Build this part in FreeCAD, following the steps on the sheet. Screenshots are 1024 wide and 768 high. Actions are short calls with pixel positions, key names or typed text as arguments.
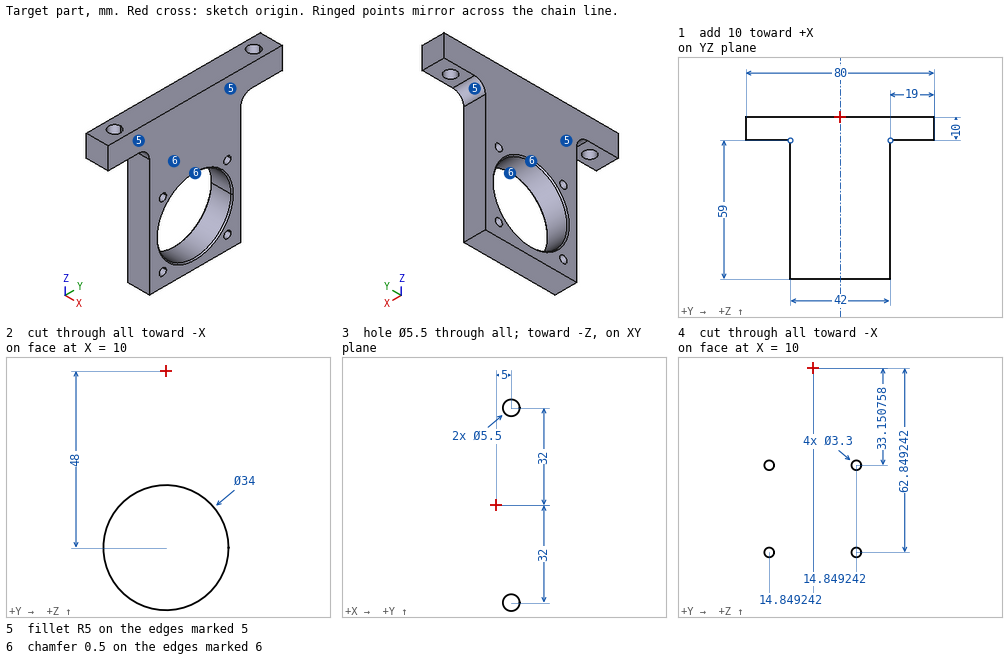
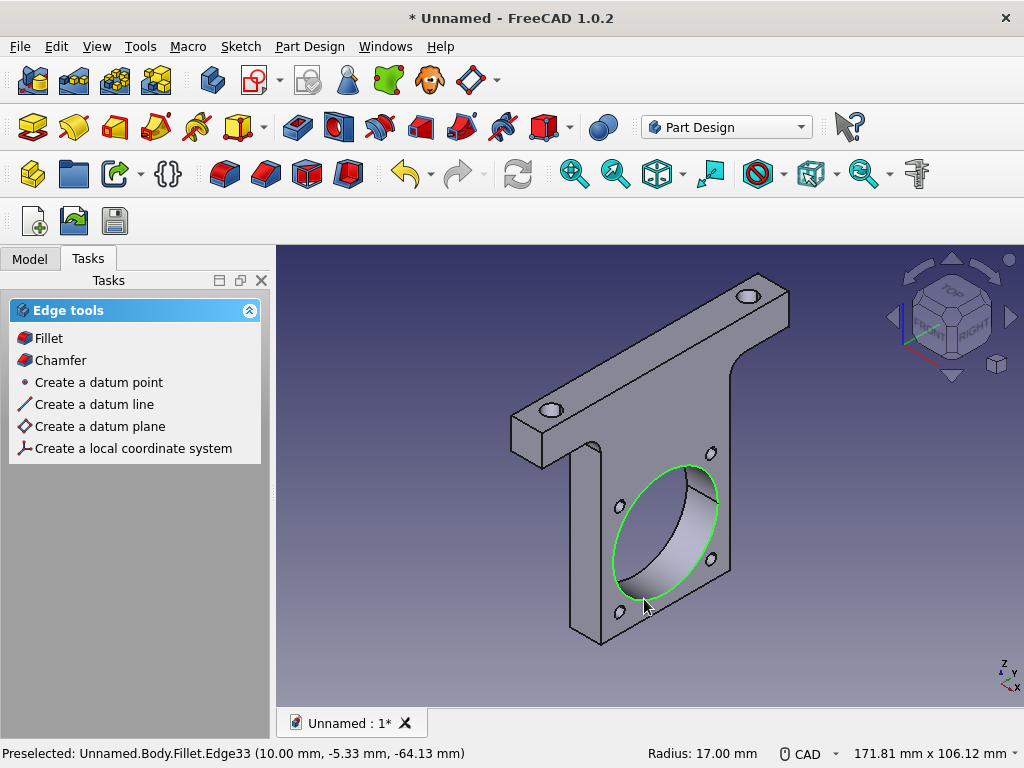
key(2)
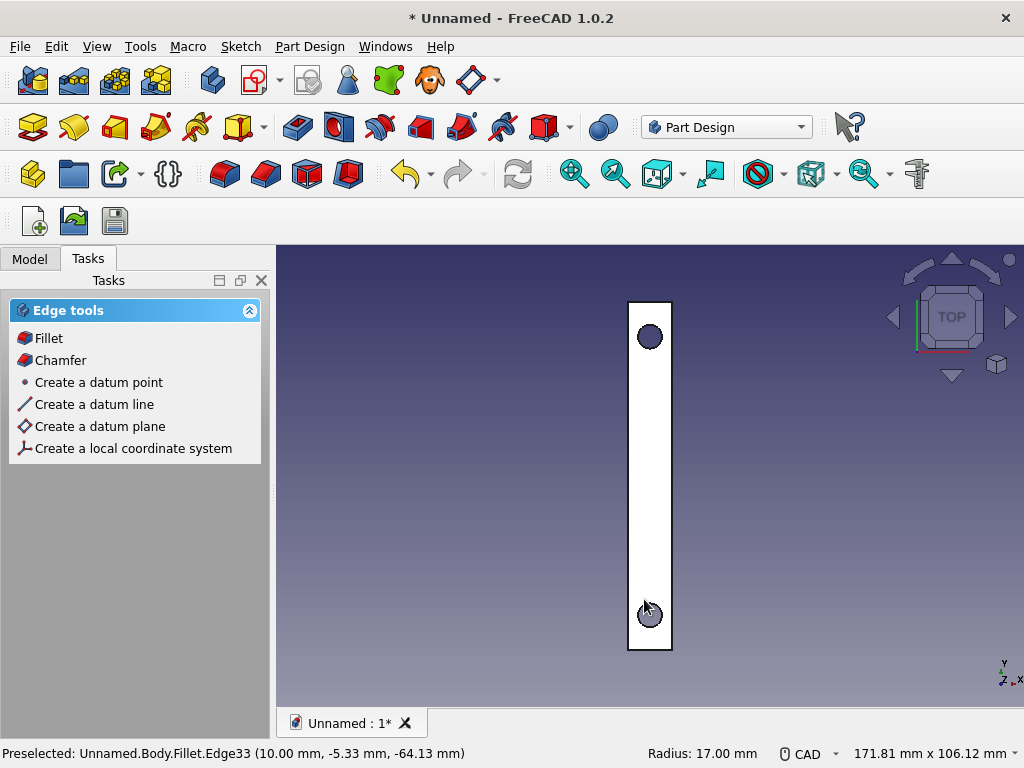
key(0)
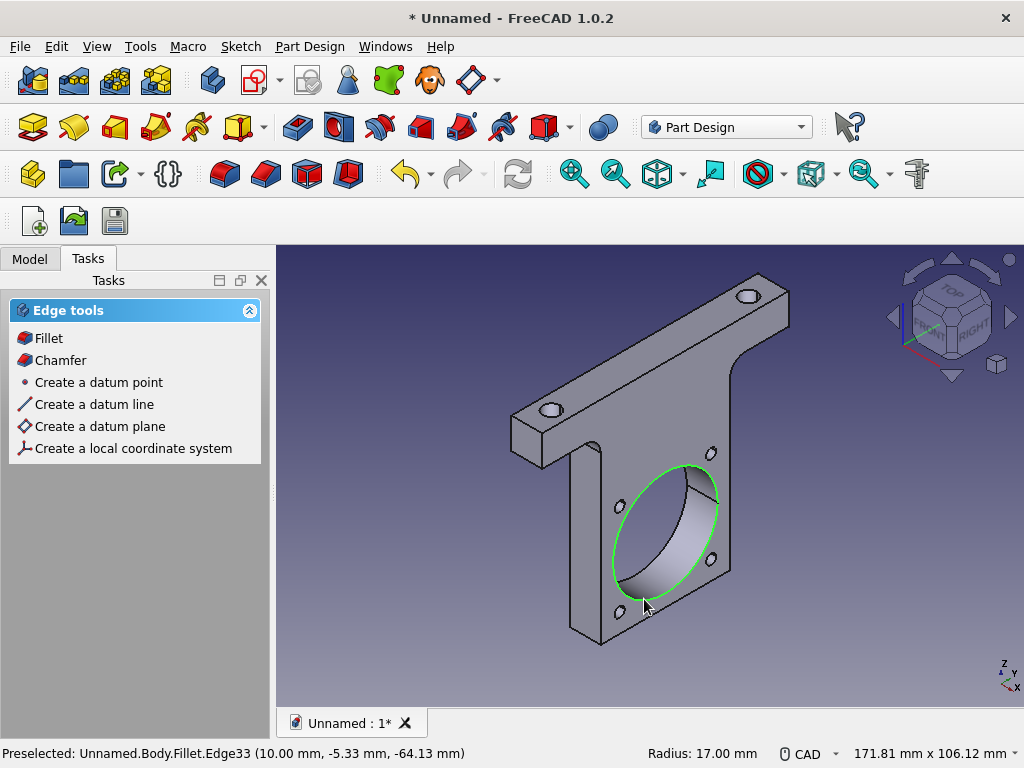
key(1)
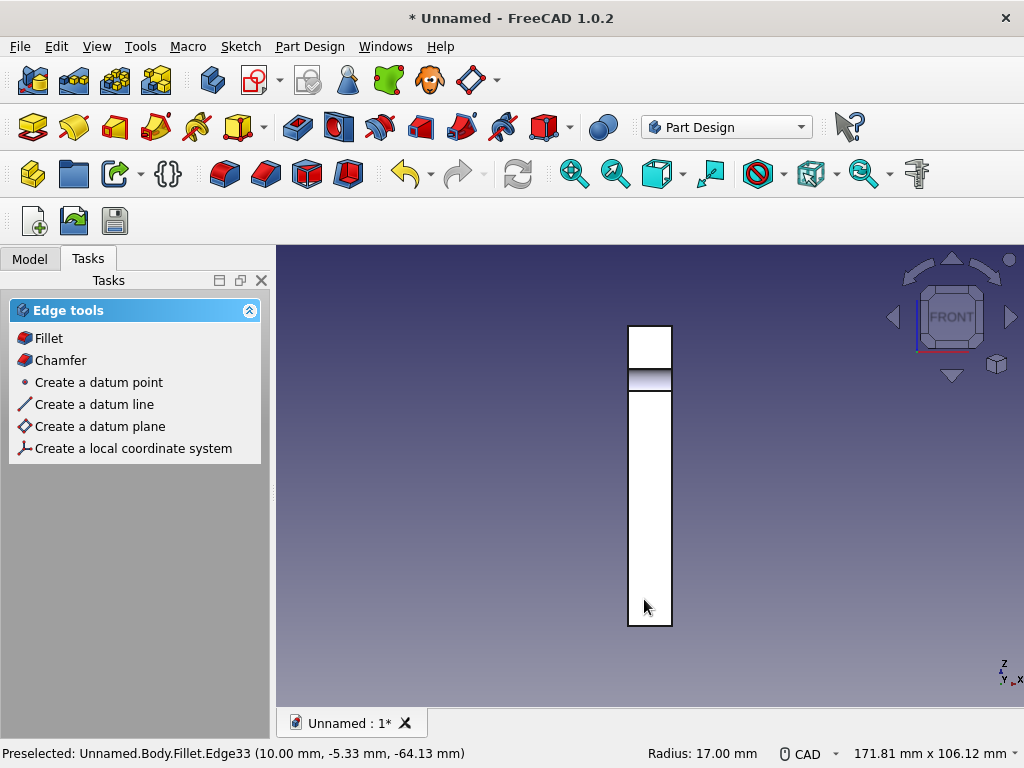
key(3)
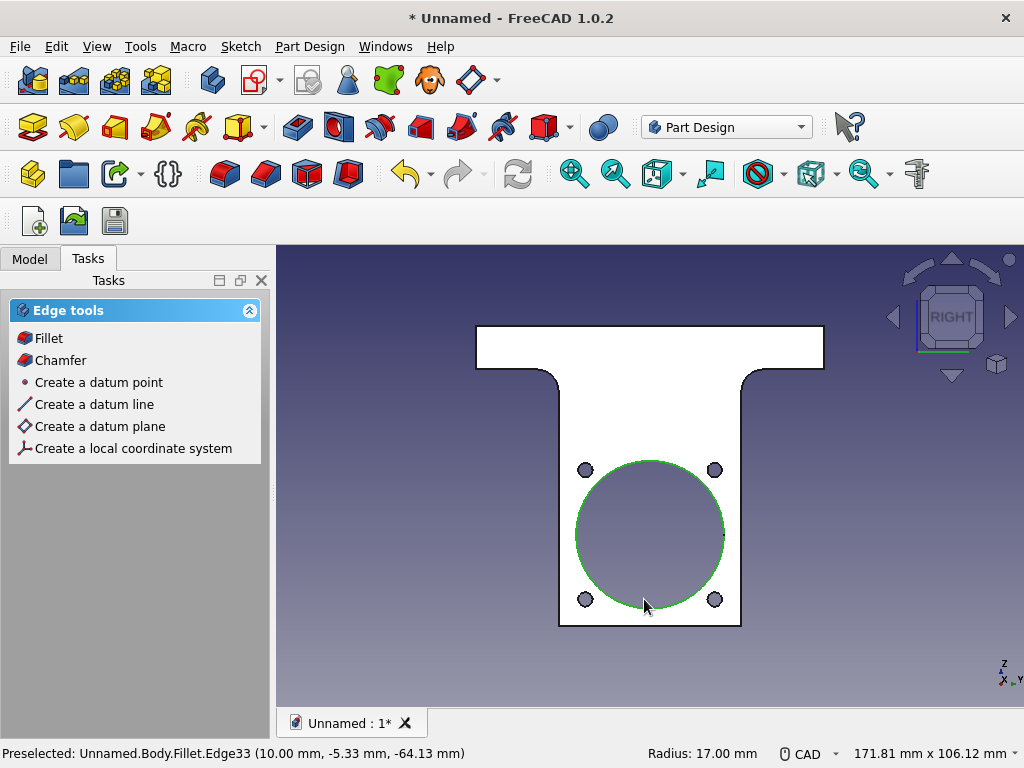
key(5)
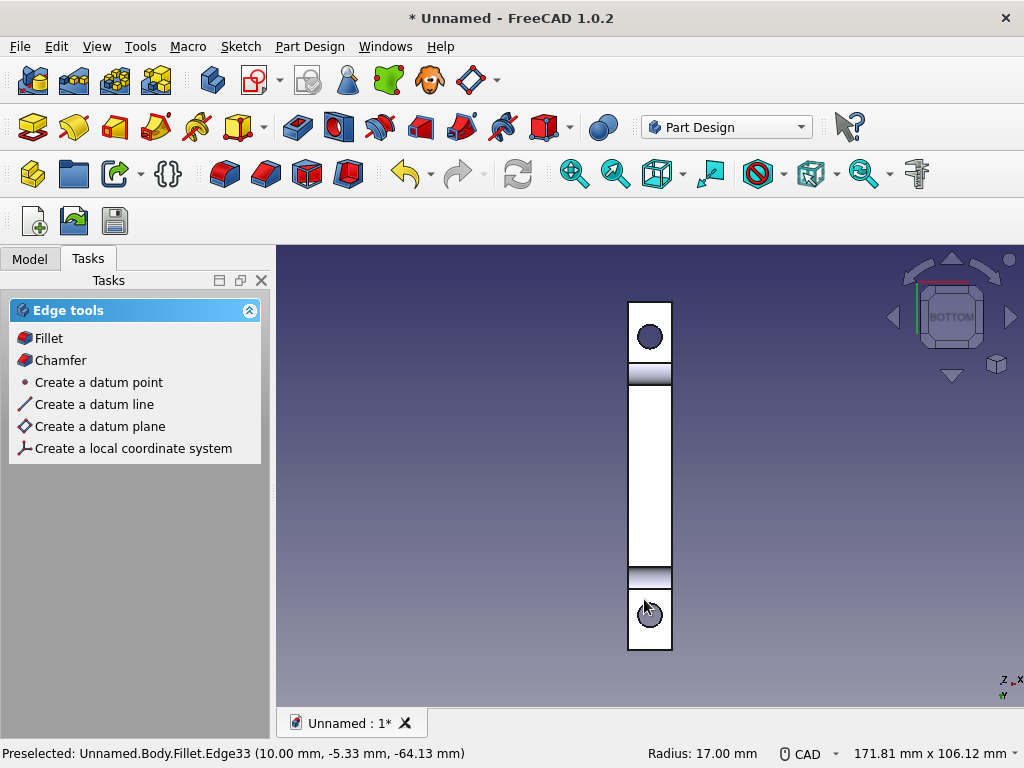
key(4)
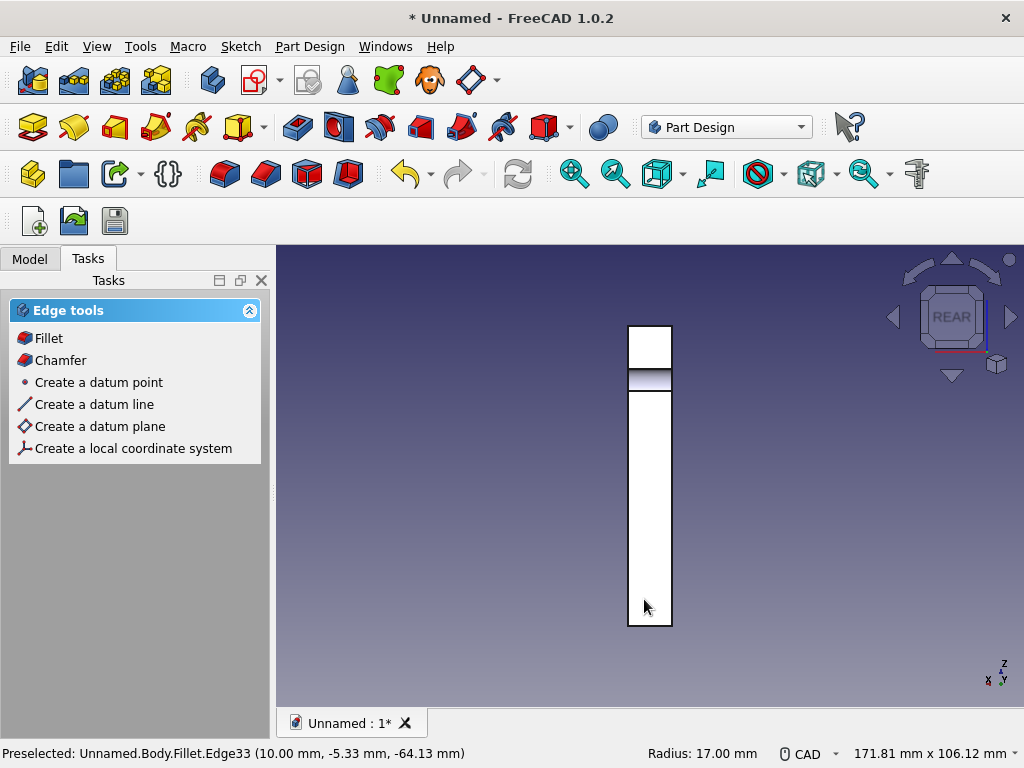
key(6)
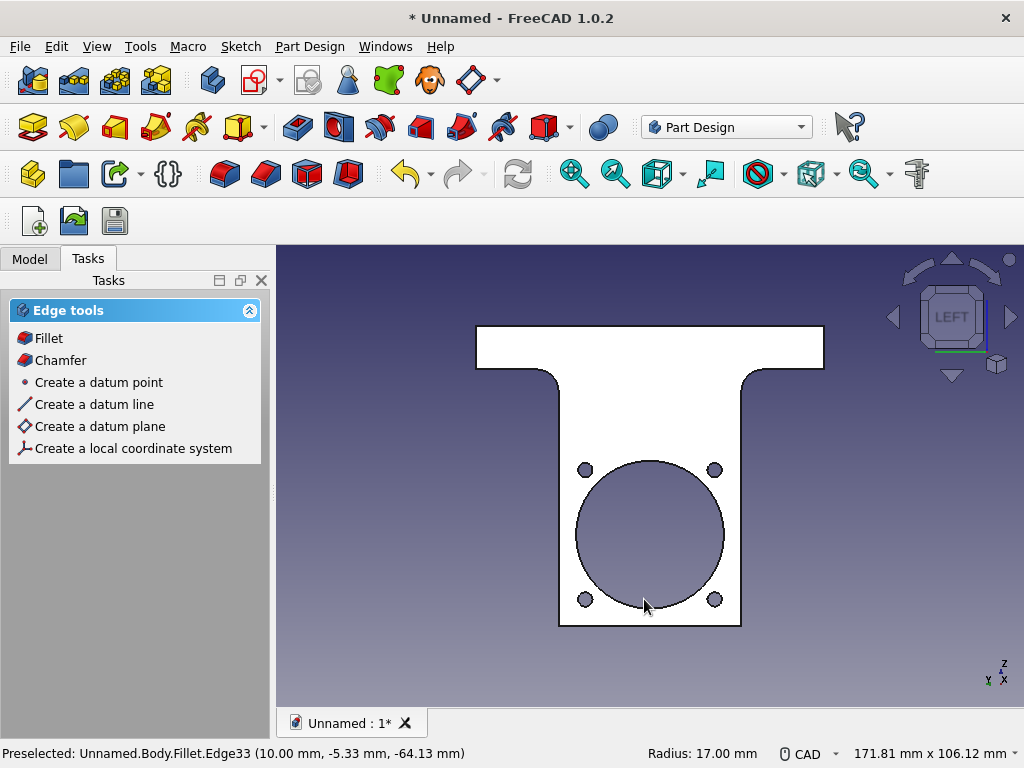
click(724, 534, ctrl)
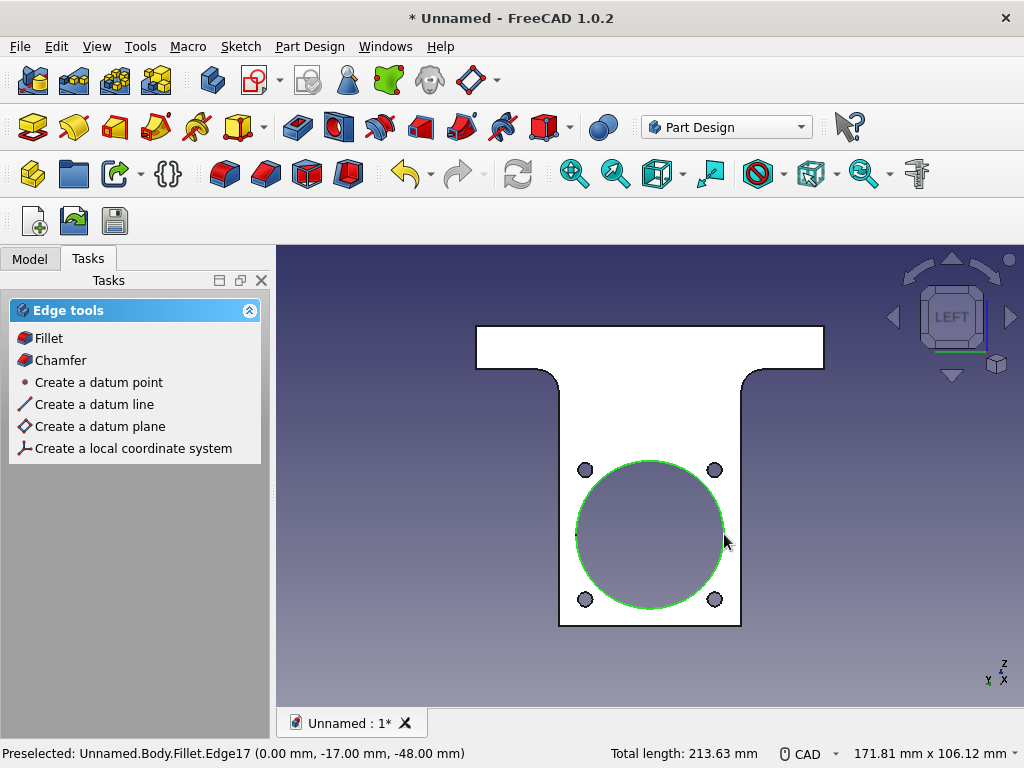
click(266, 174)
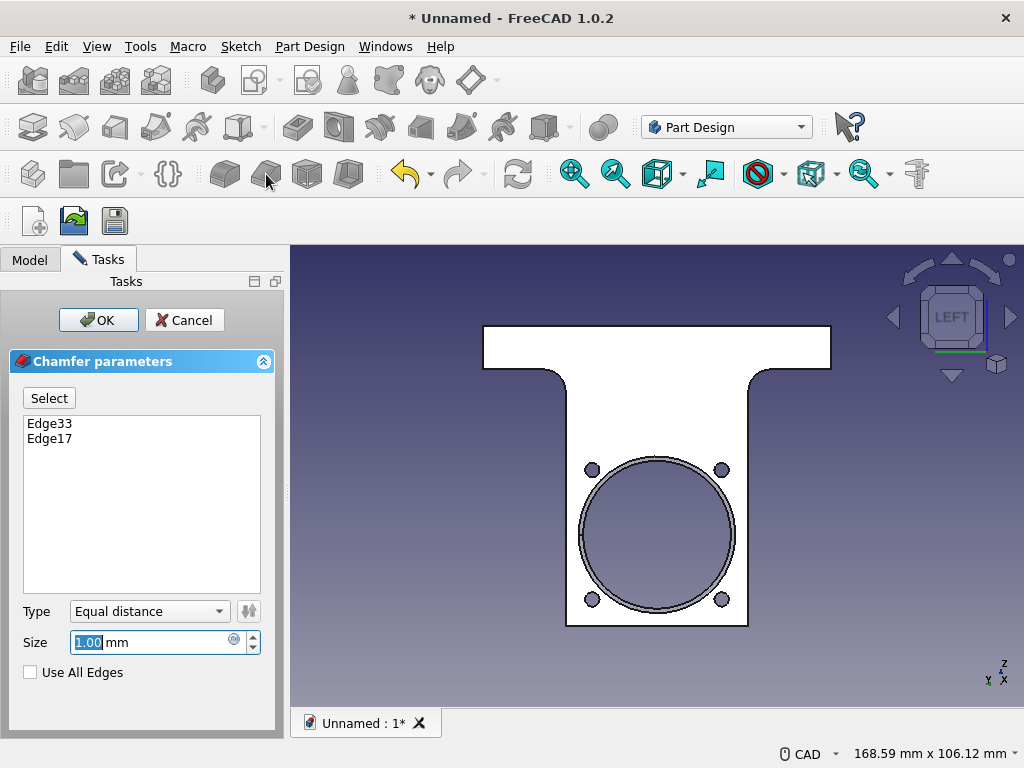
text(0.5)
key(Tab)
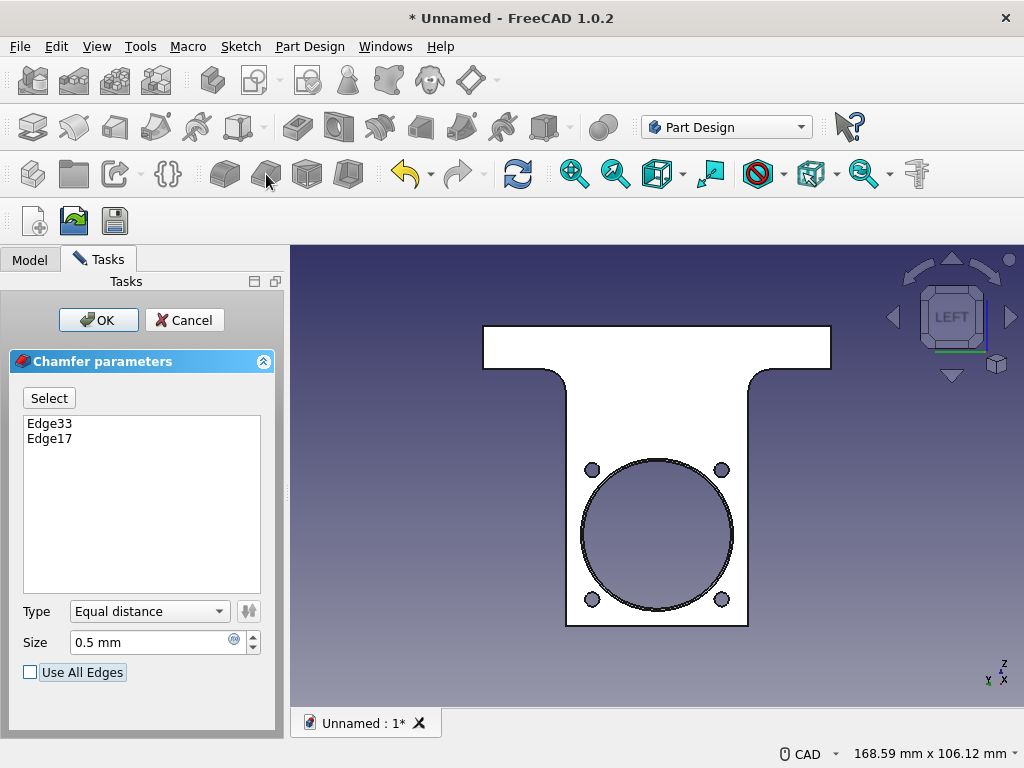
click(99, 320)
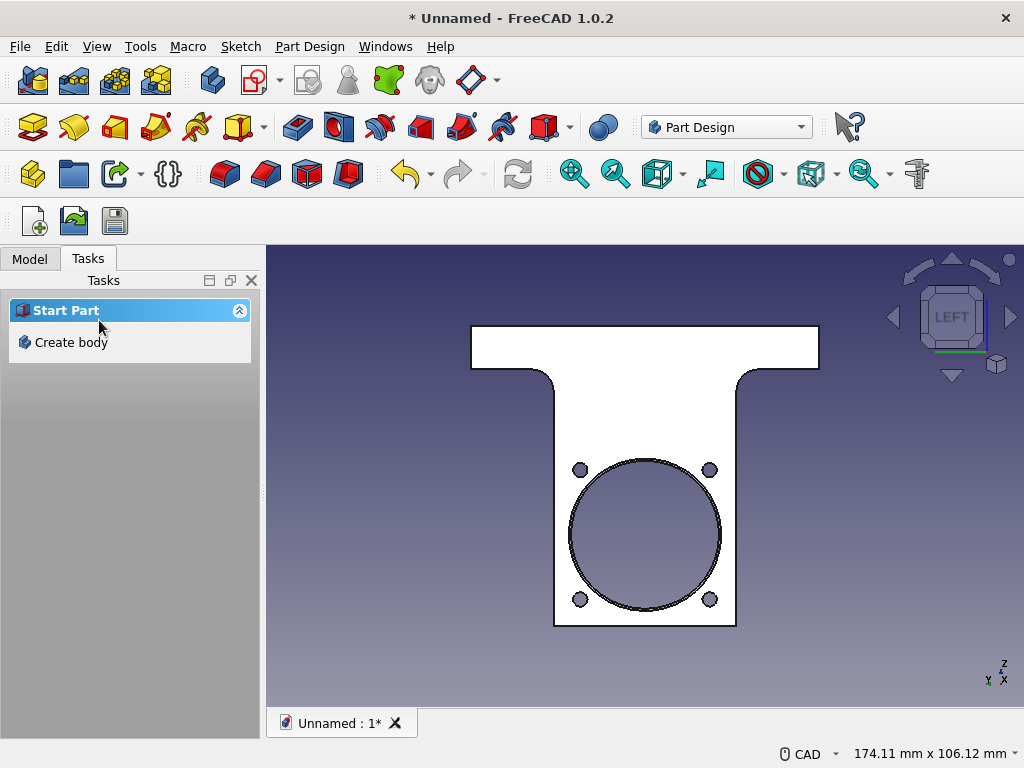
key(0)